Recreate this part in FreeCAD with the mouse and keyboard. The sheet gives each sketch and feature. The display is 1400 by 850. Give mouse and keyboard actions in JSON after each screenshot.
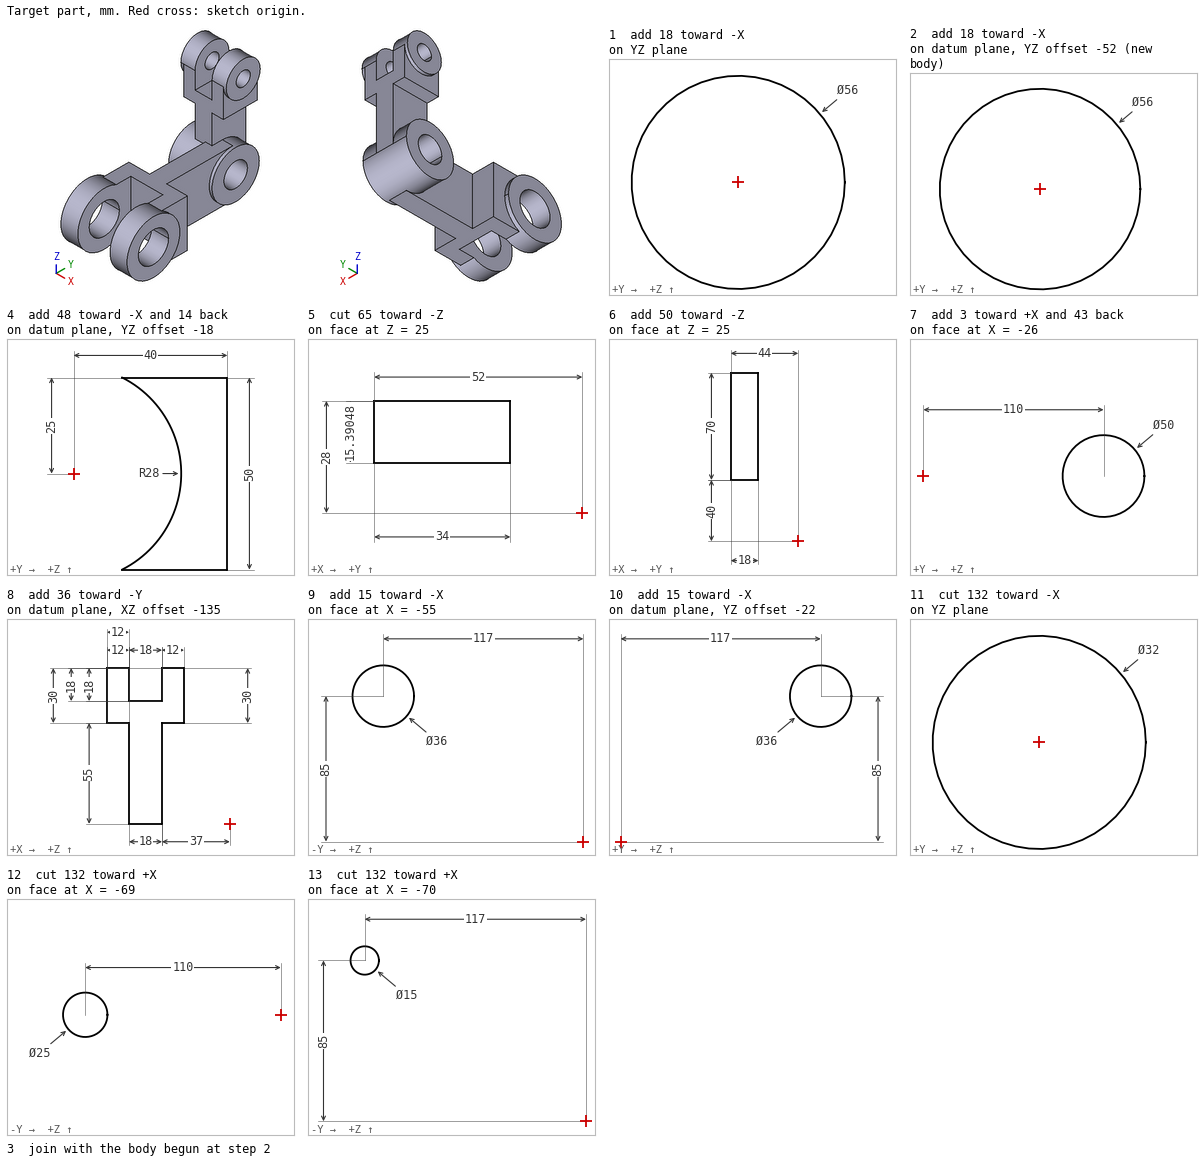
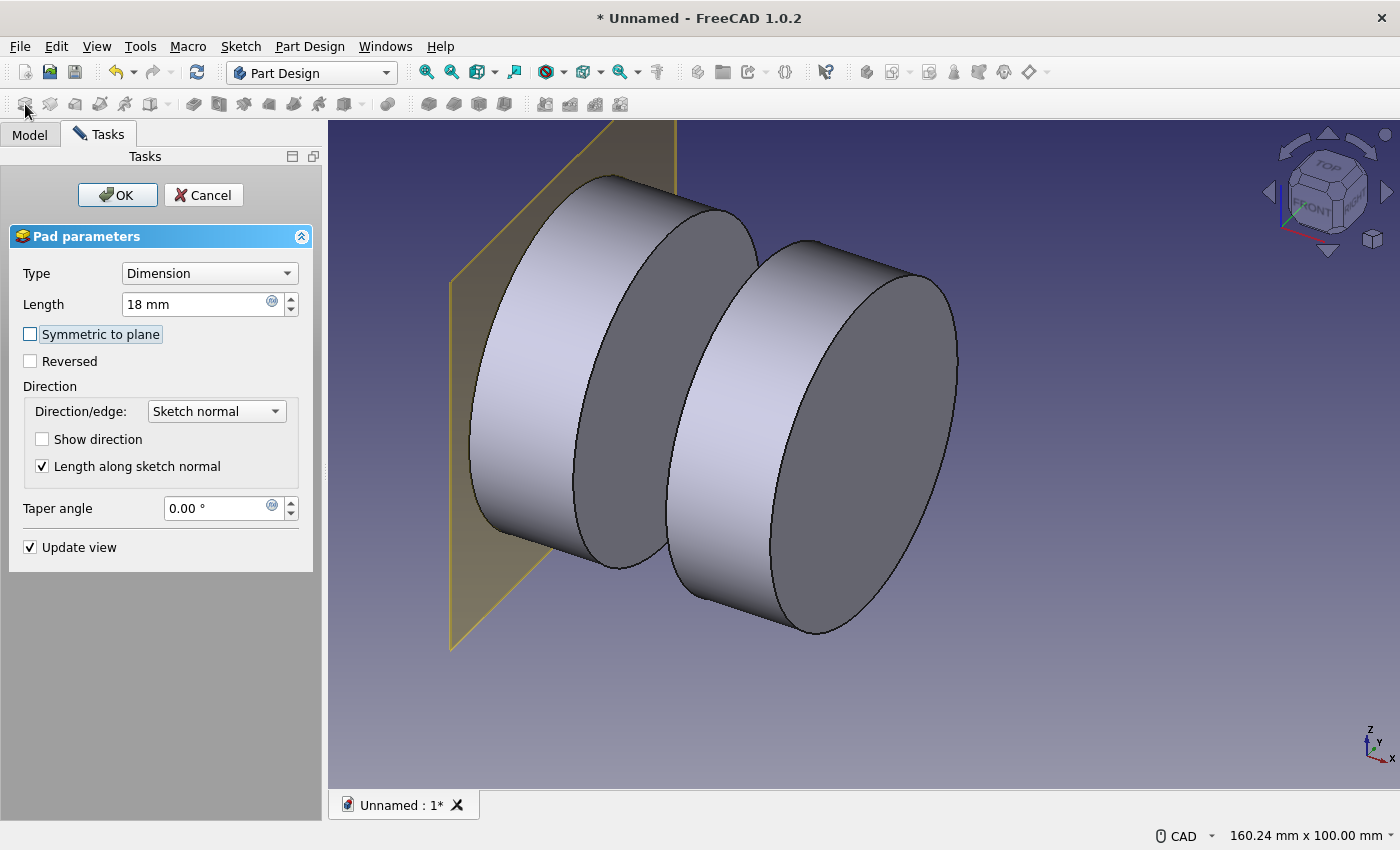
{"action": "left_click", "coordinate": [31, 361]}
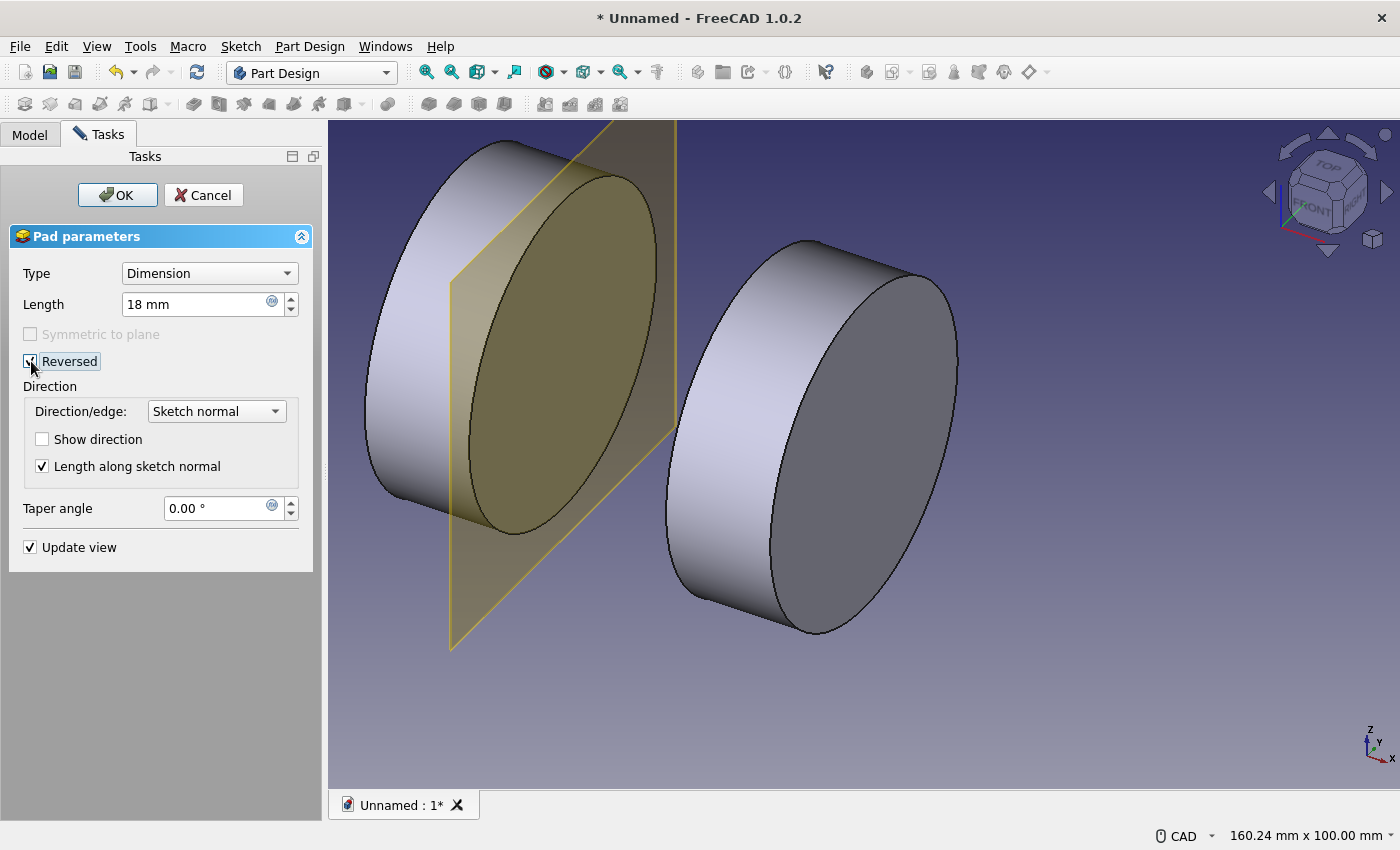
{"action": "left_click", "coordinate": [118, 195]}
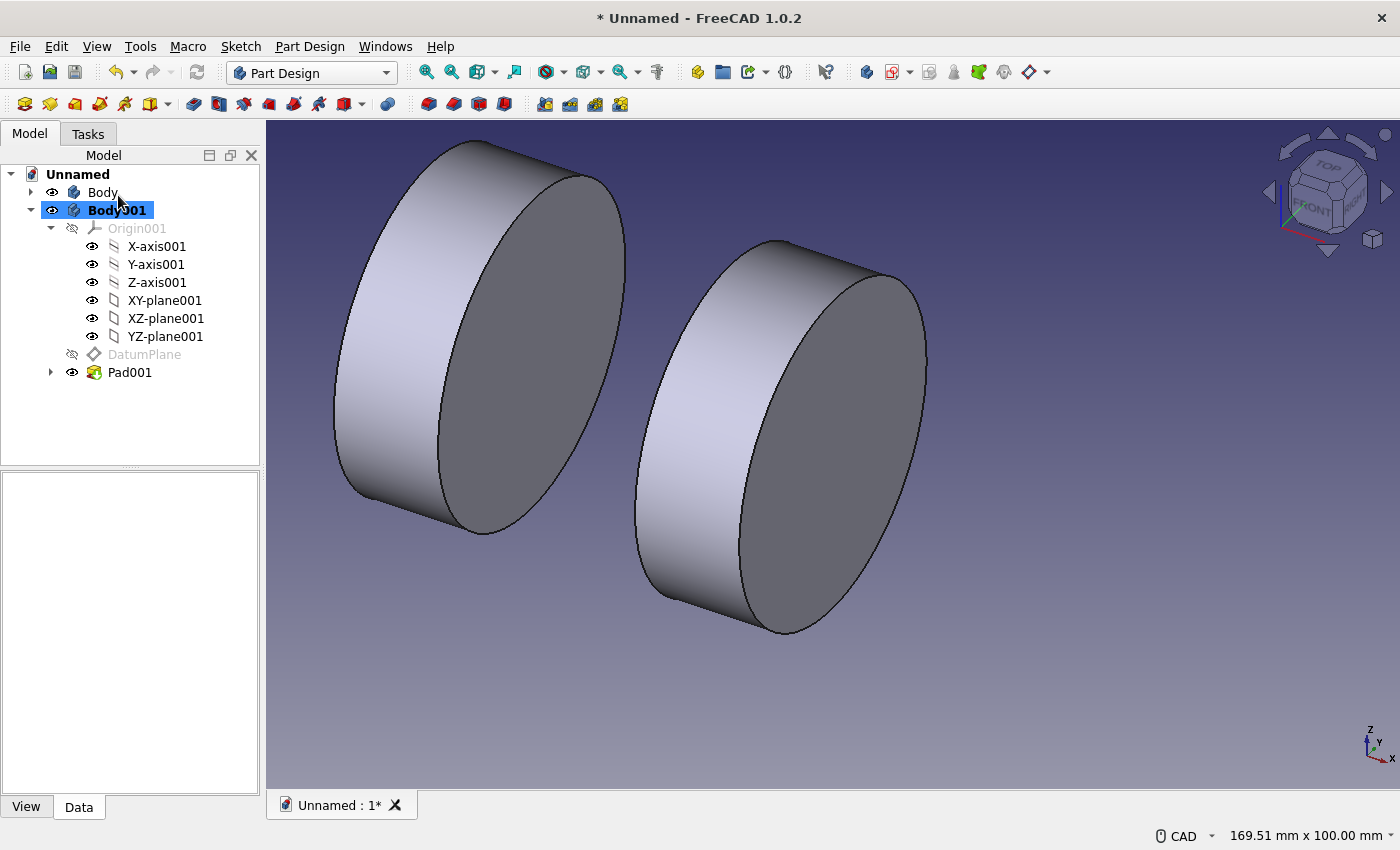
{"action": "left_click", "coordinate": [427, 72]}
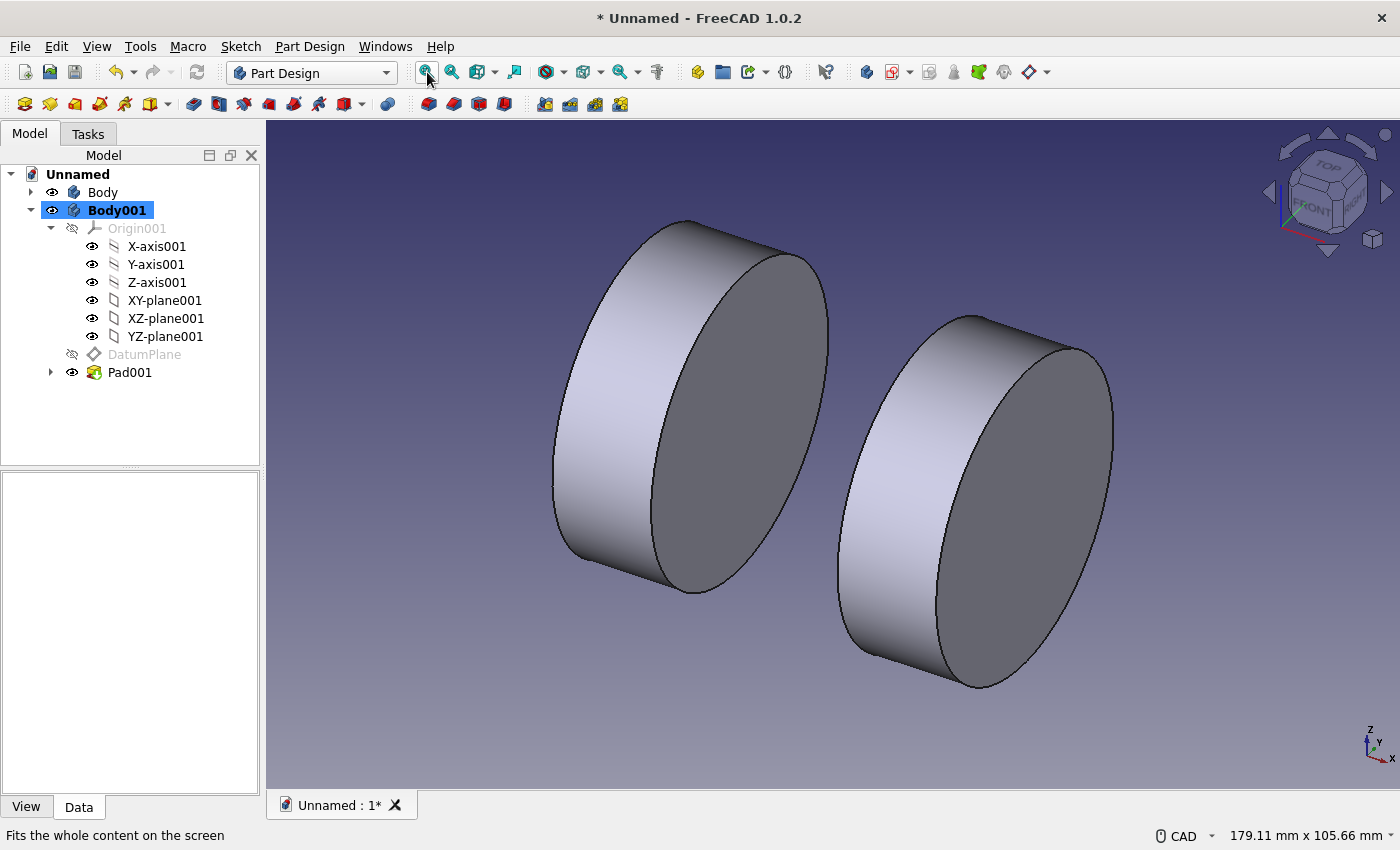
{"action": "double_click", "coordinate": [97, 192]}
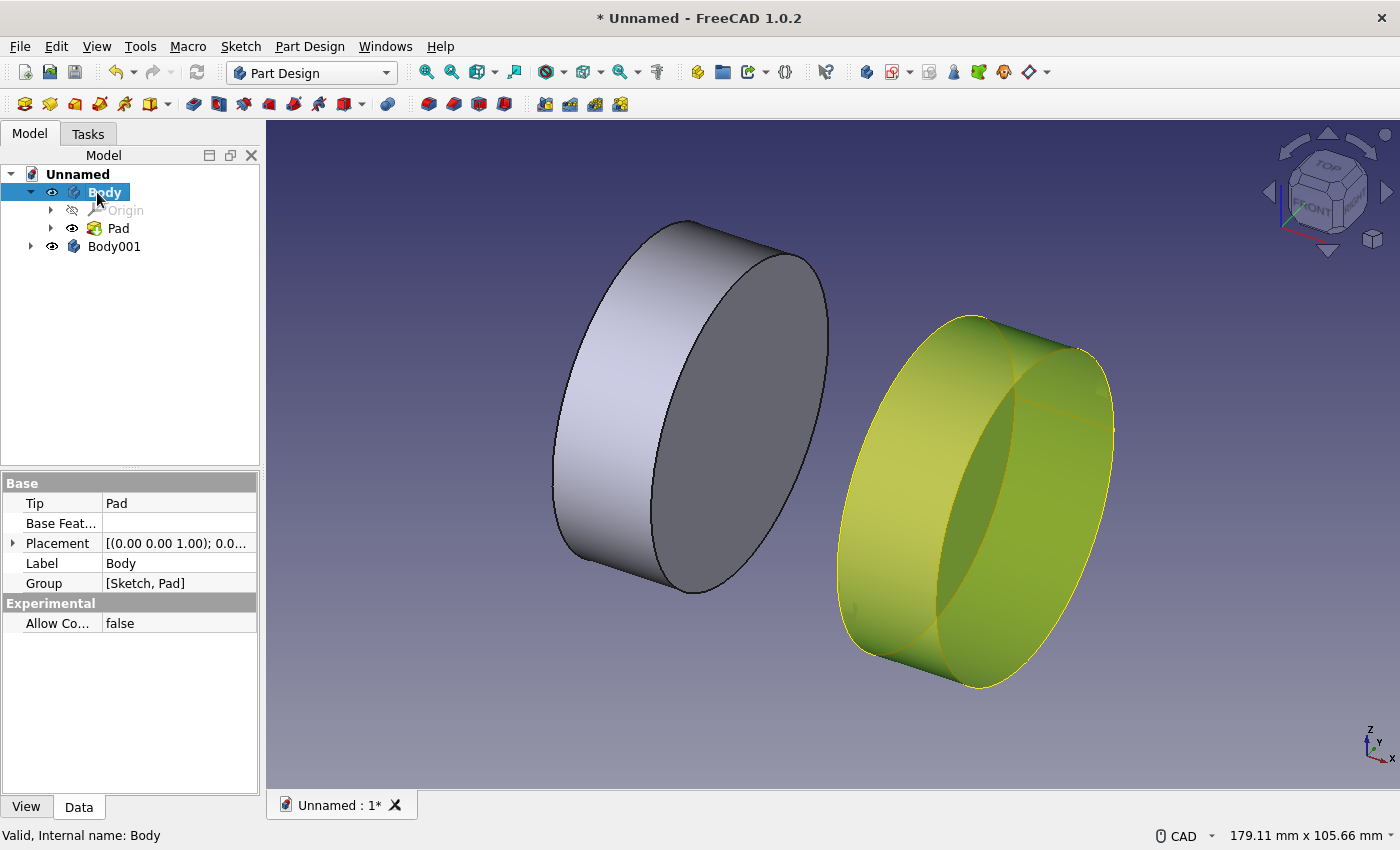
{"action": "left_click", "coordinate": [97, 192]}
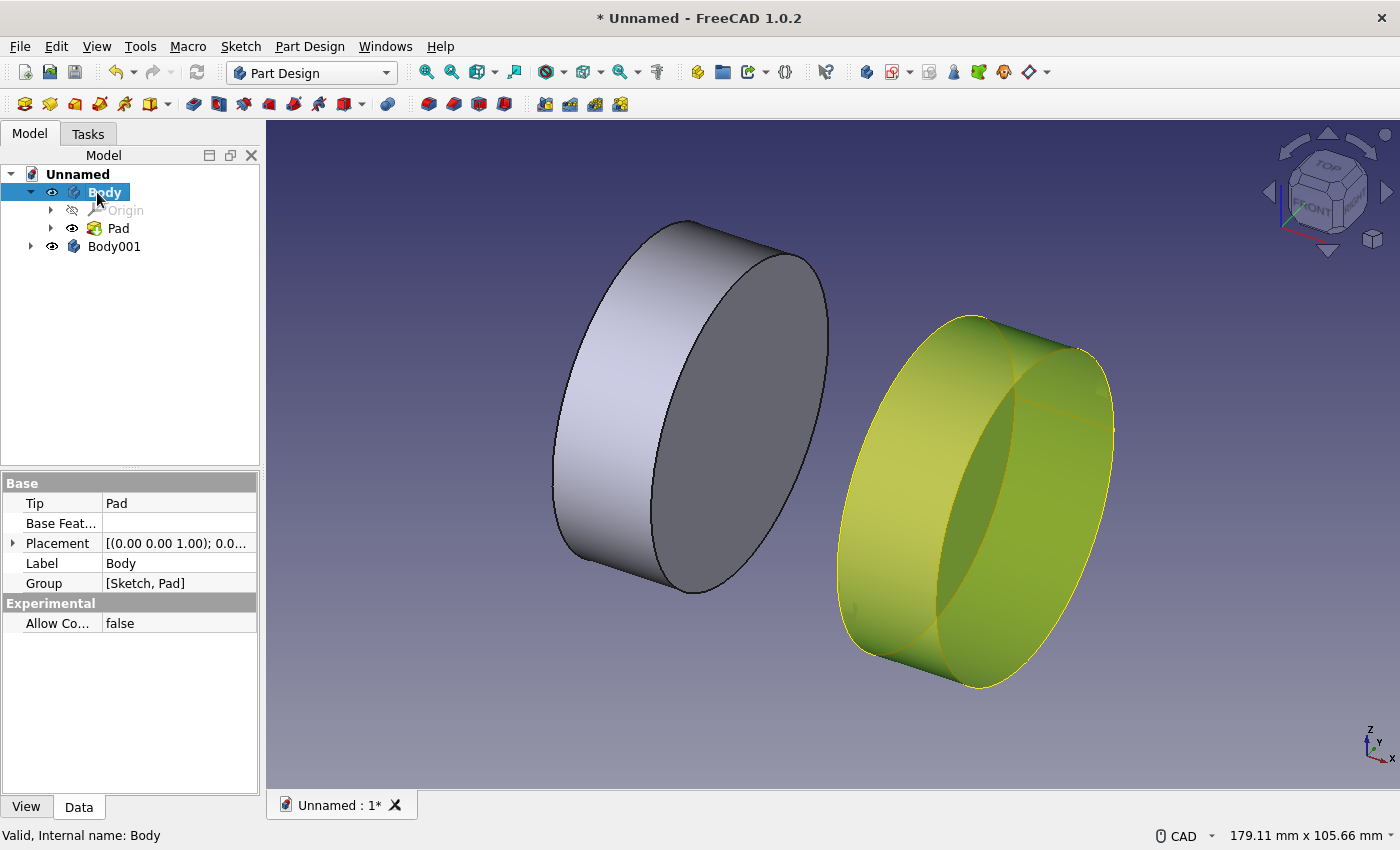
{"action": "left_click", "coordinate": [148, 623]}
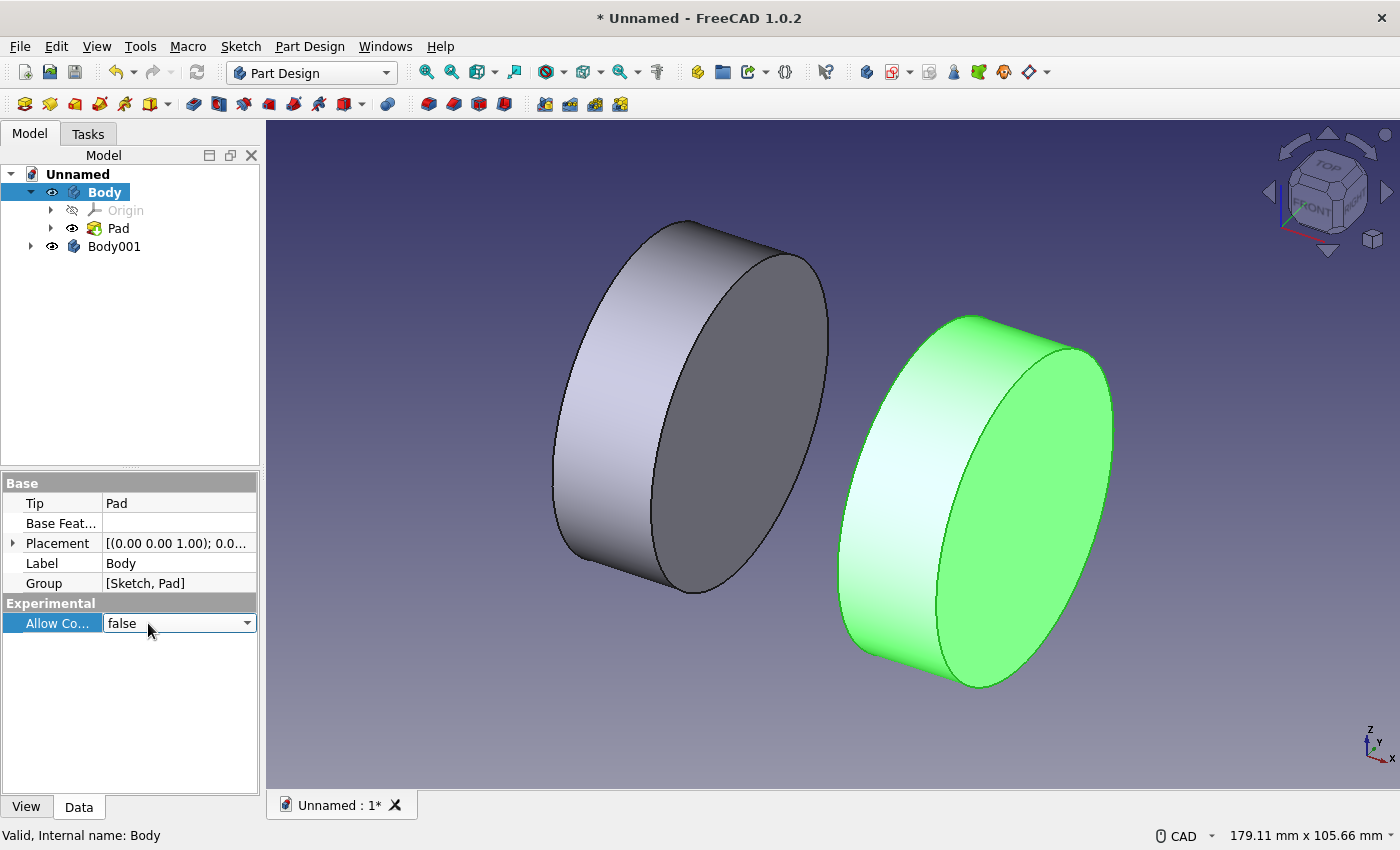
{"action": "left_click", "coordinate": [148, 623]}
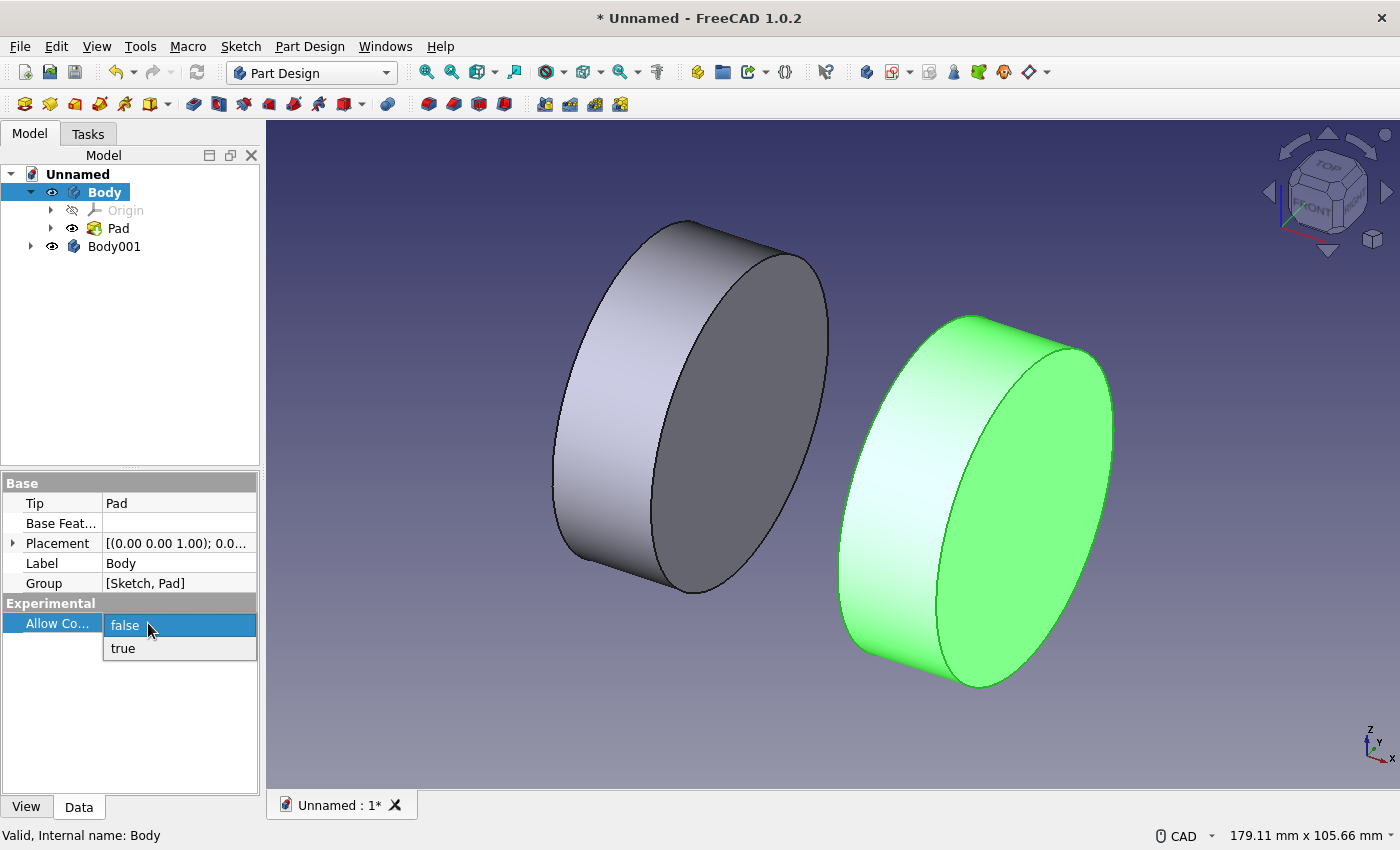
{"action": "left_click", "coordinate": [178, 648]}
{"action": "key", "text": "Return"}